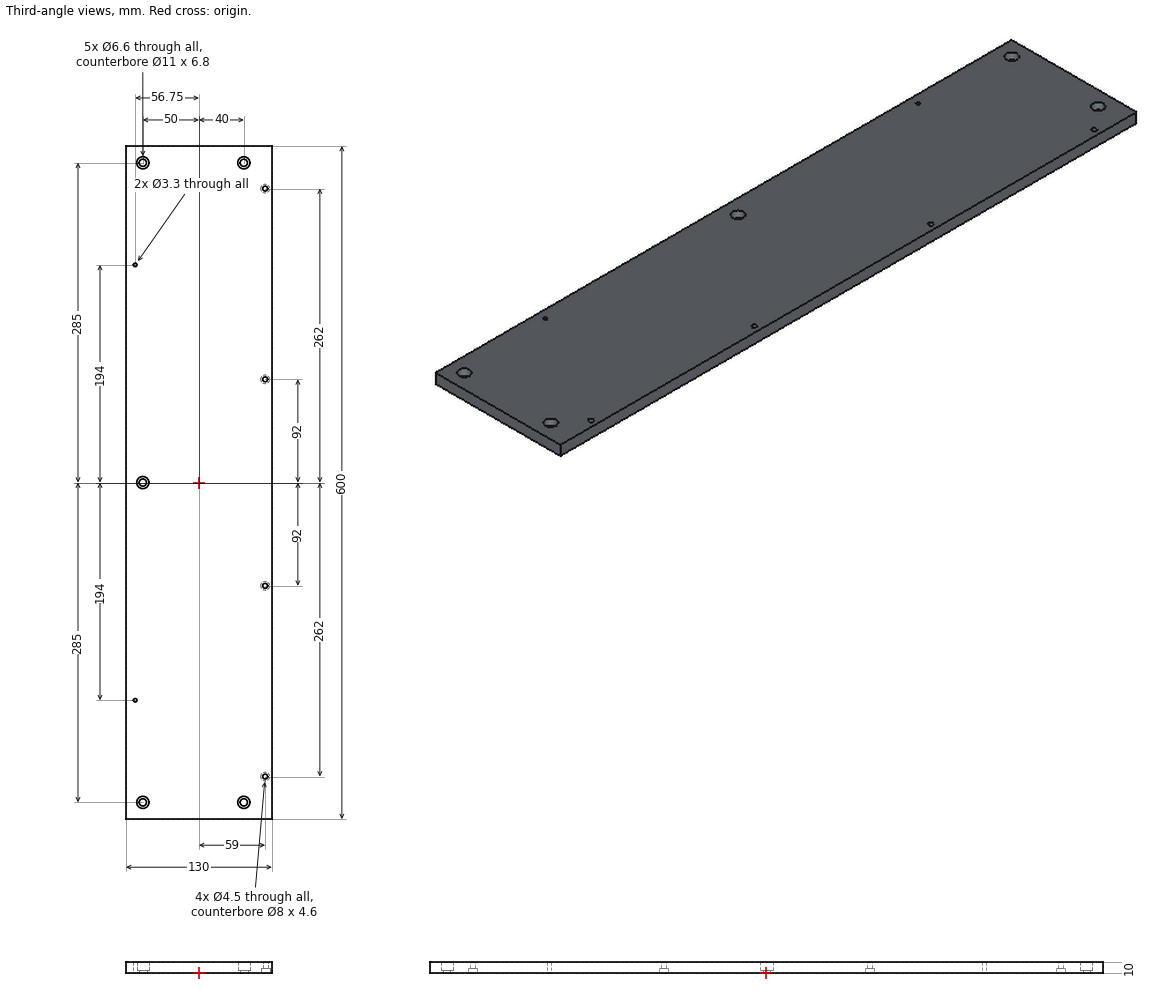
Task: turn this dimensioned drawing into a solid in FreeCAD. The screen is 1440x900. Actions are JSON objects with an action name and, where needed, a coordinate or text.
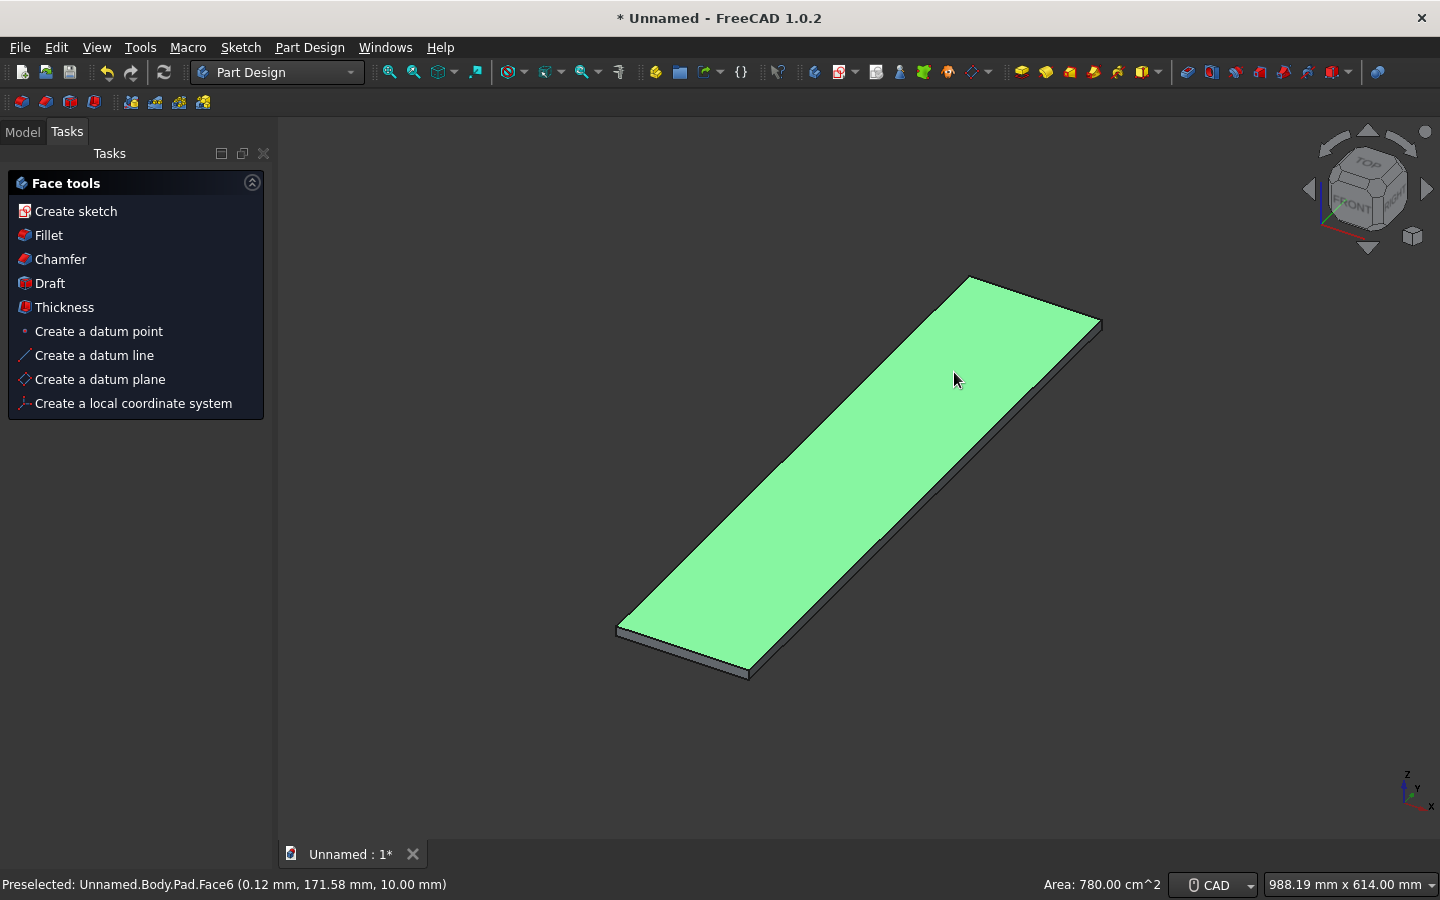
{"action": "left_click", "coordinate": [840, 72]}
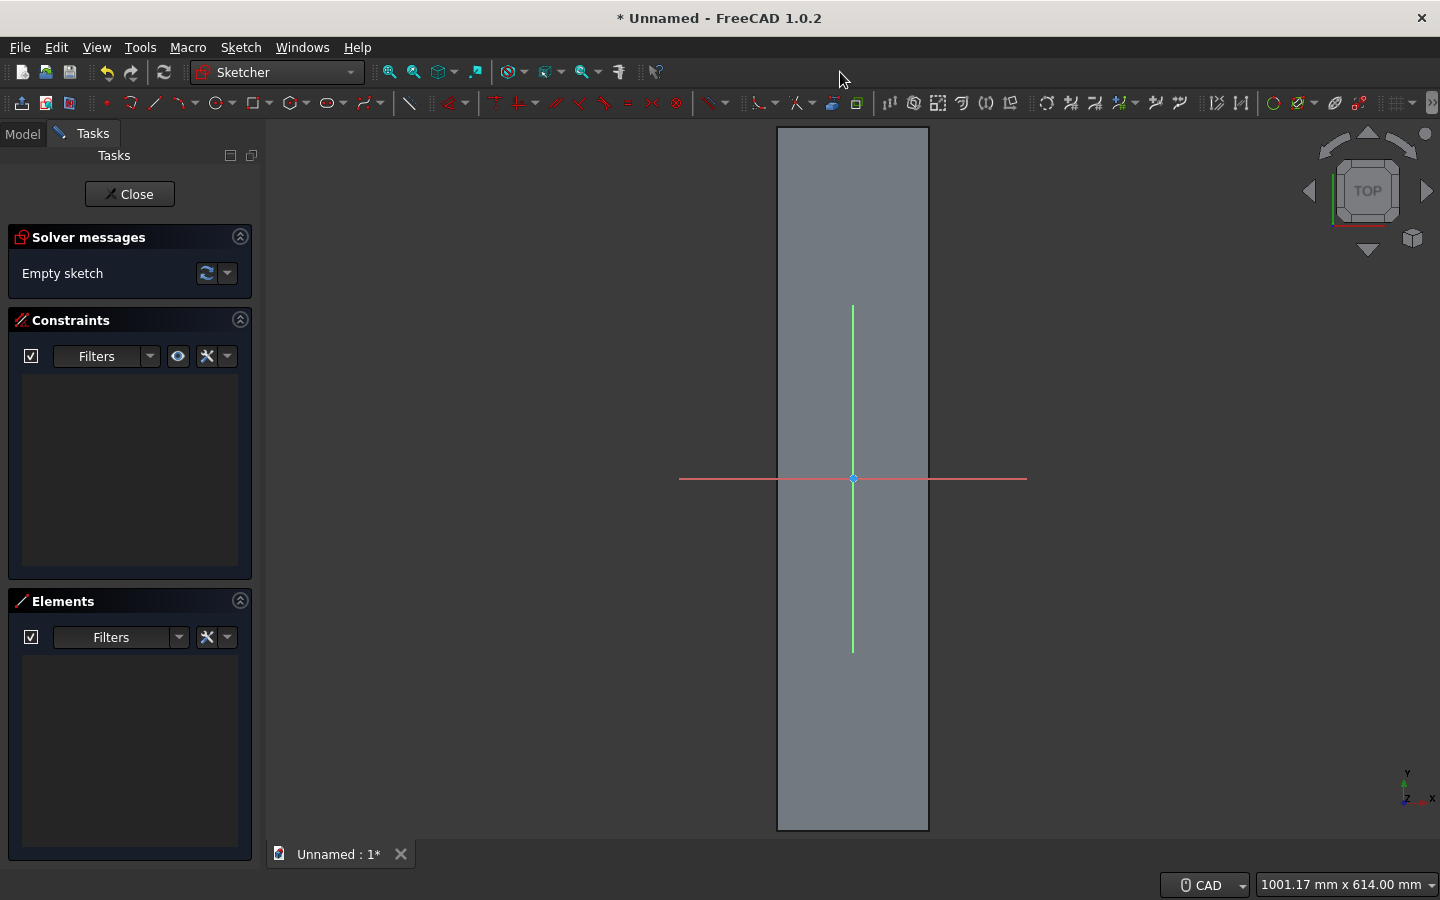
{"action": "scroll", "coordinate": [657, 479], "scroll_direction": "down", "scroll_amount": 2}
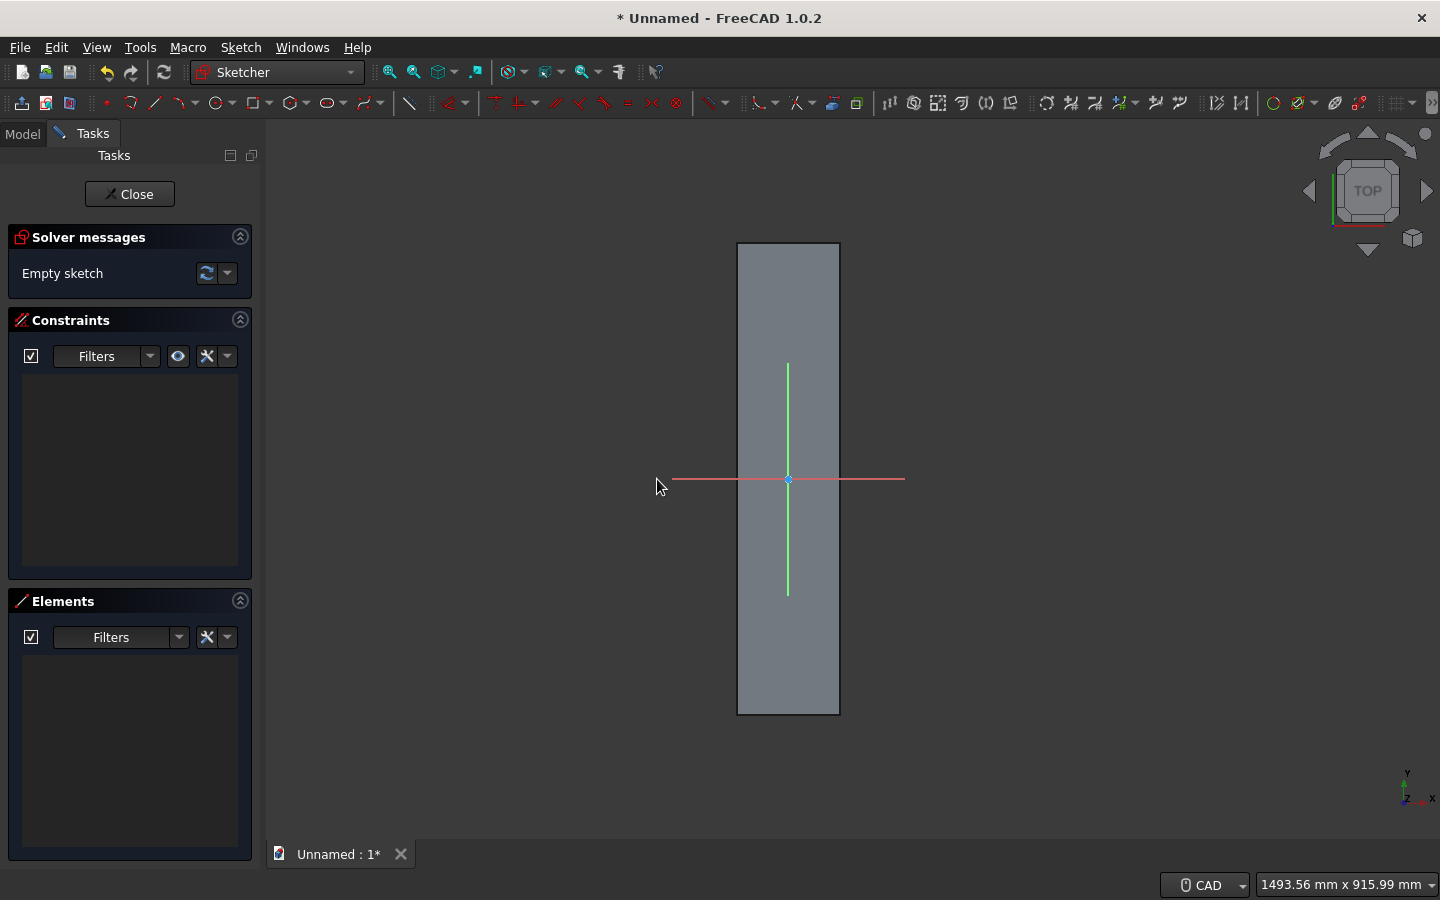
{"action": "left_click", "coordinate": [216, 104]}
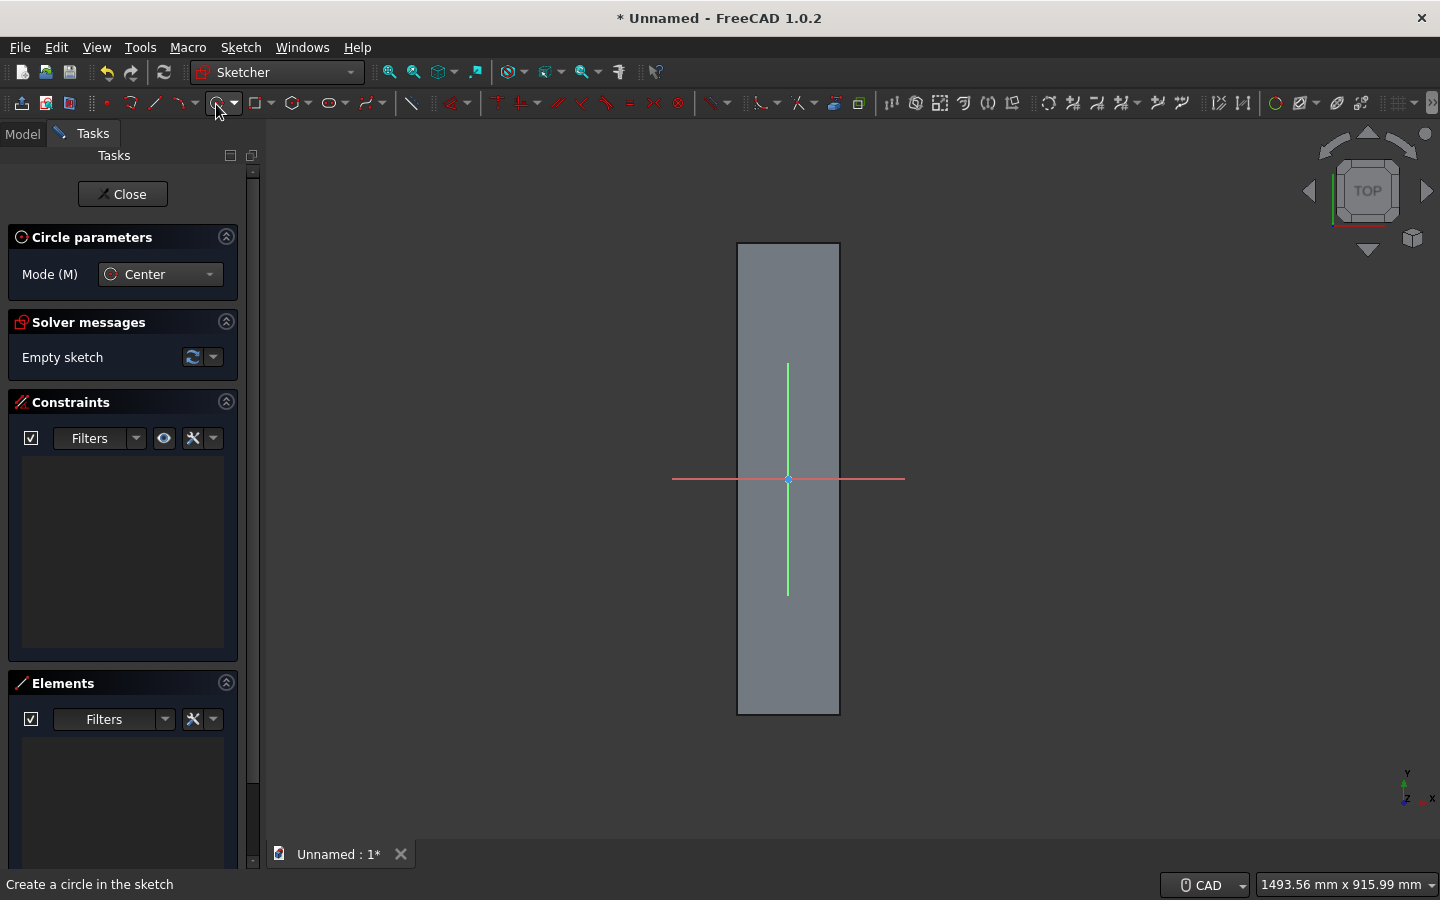
{"action": "scroll", "coordinate": [749, 255], "scroll_direction": "up", "scroll_amount": 11}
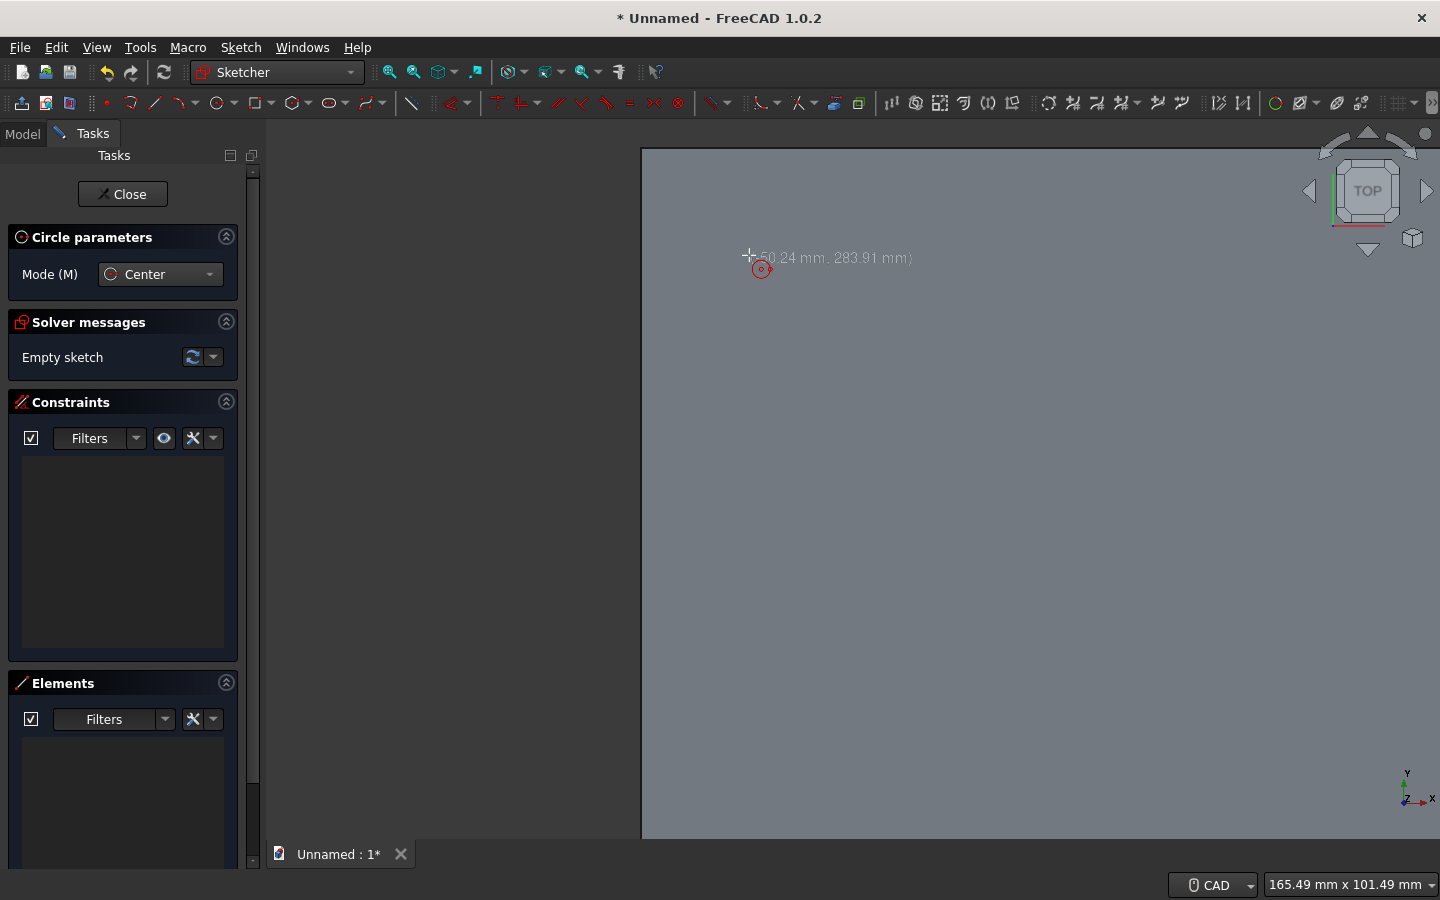
{"action": "scroll", "coordinate": [749, 255], "scroll_direction": "down", "scroll_amount": 11}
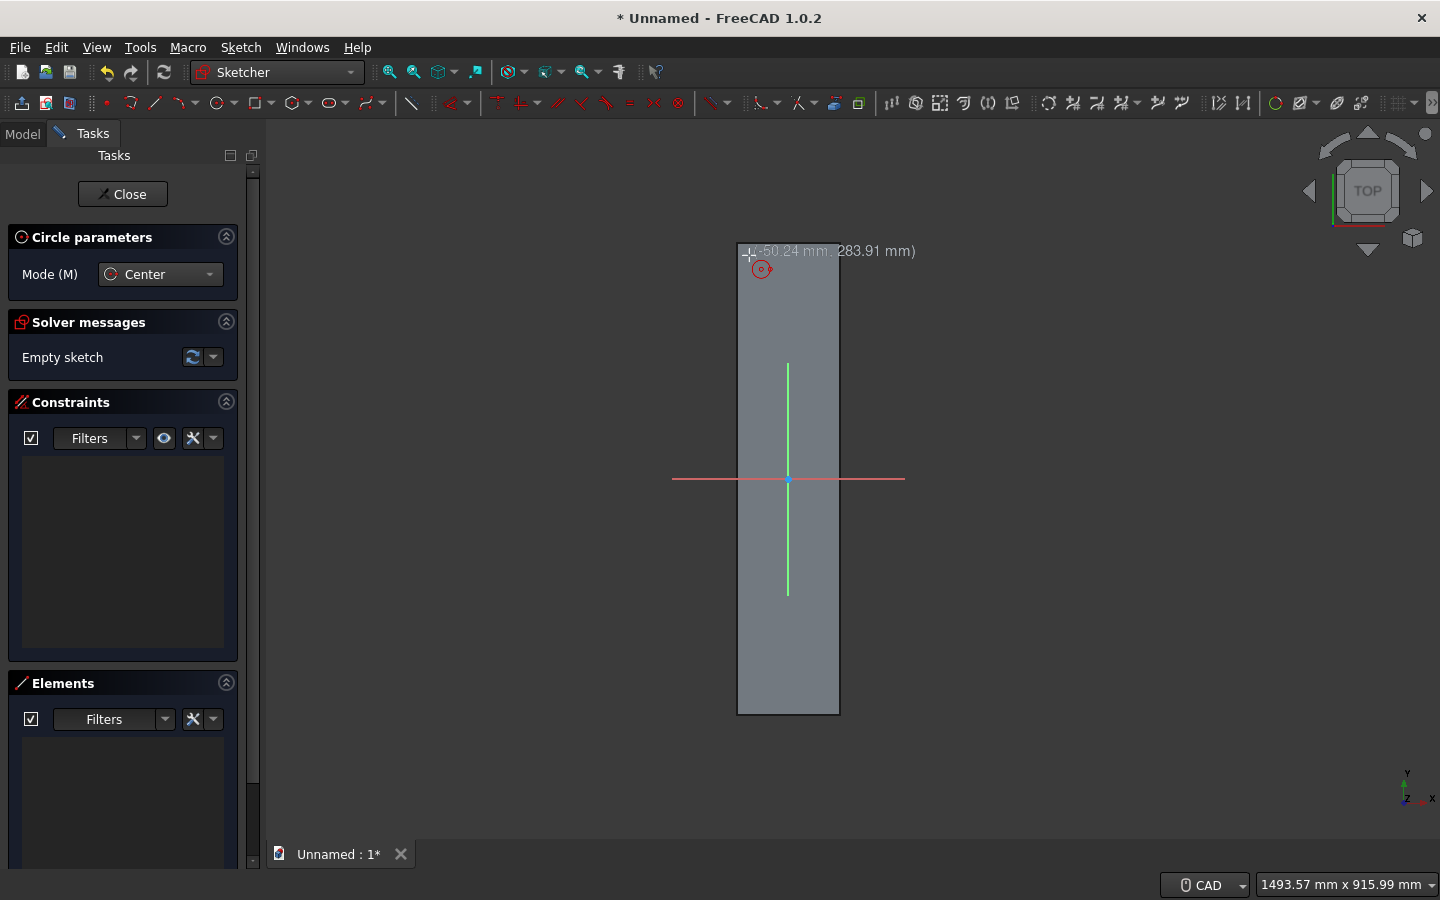
{"action": "left_click", "coordinate": [749, 255]}
{"action": "mouse_move", "coordinate": [751, 253]}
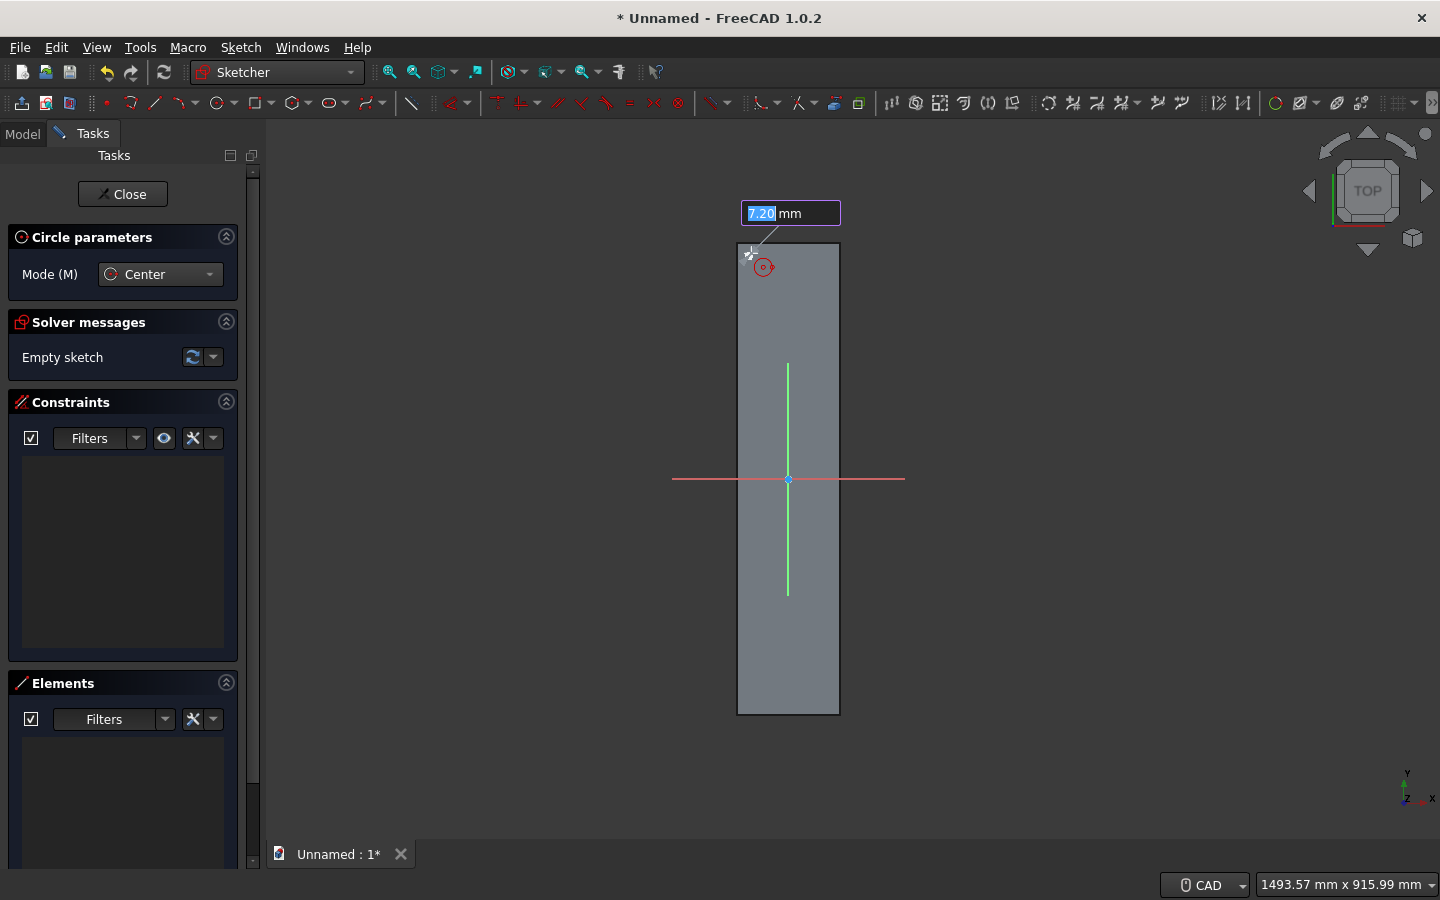
{"action": "type", "text": "6.6"}
{"action": "key", "text": "Return"}